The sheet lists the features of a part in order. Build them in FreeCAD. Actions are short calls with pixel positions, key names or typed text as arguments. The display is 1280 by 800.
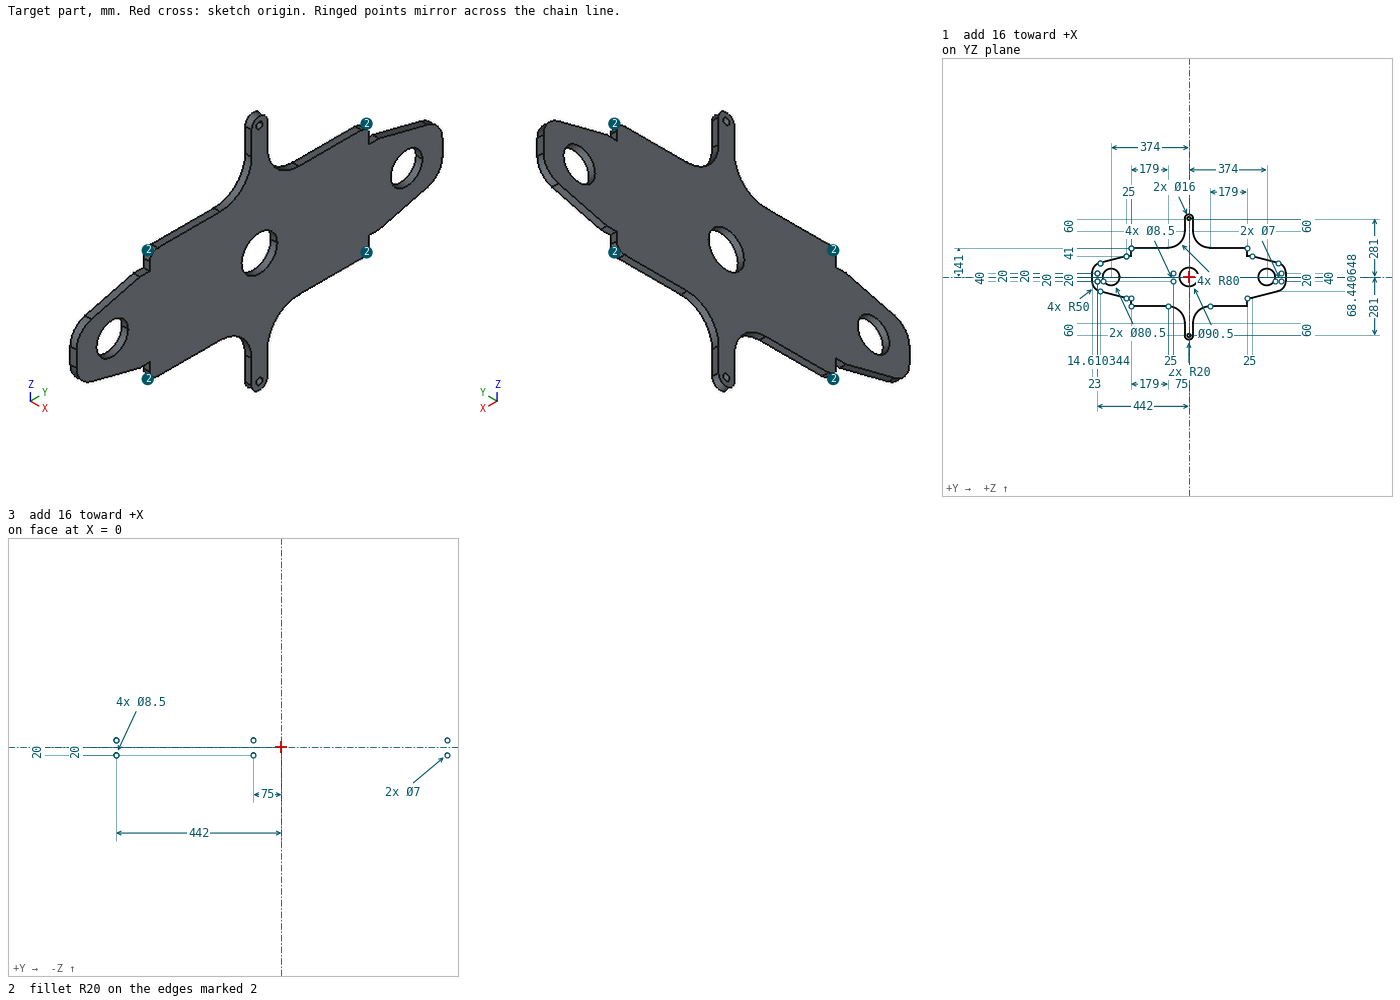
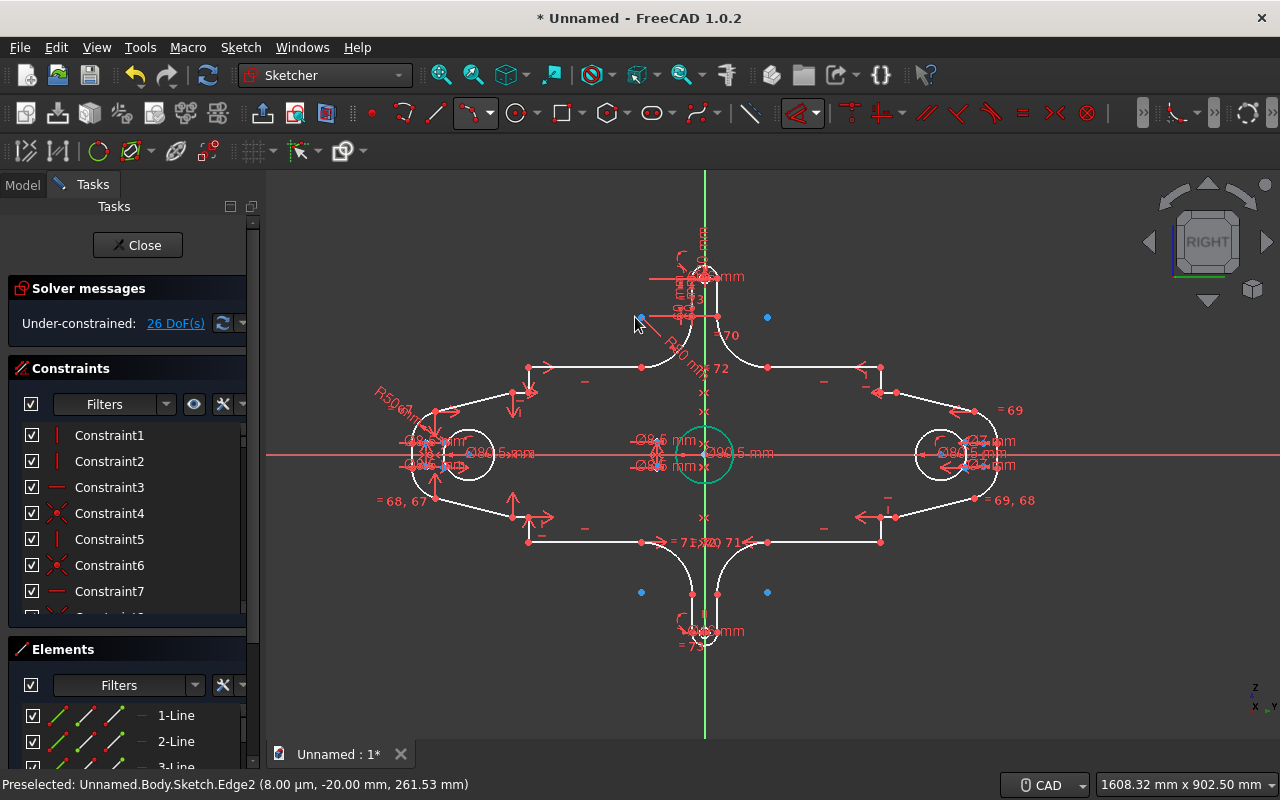
scroll(529, 375, up, 4)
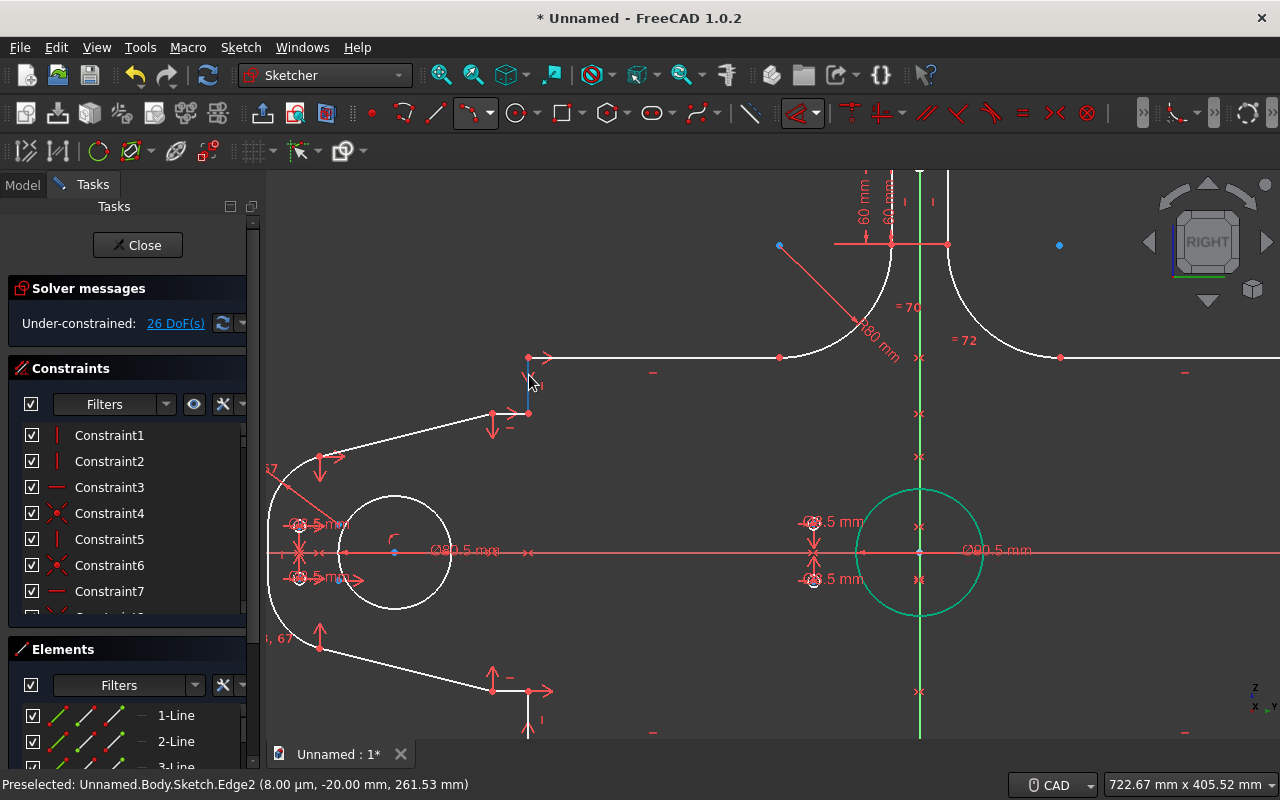
click(528, 375)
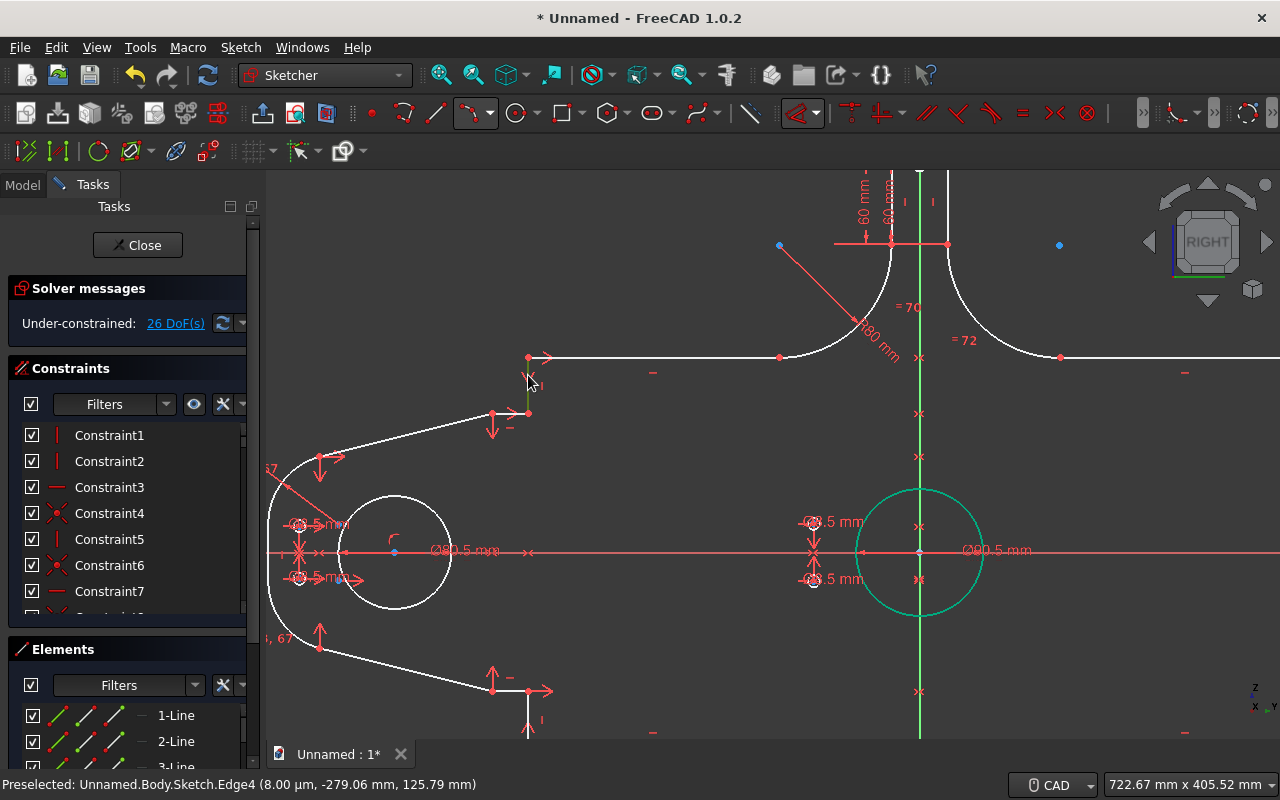
key(i)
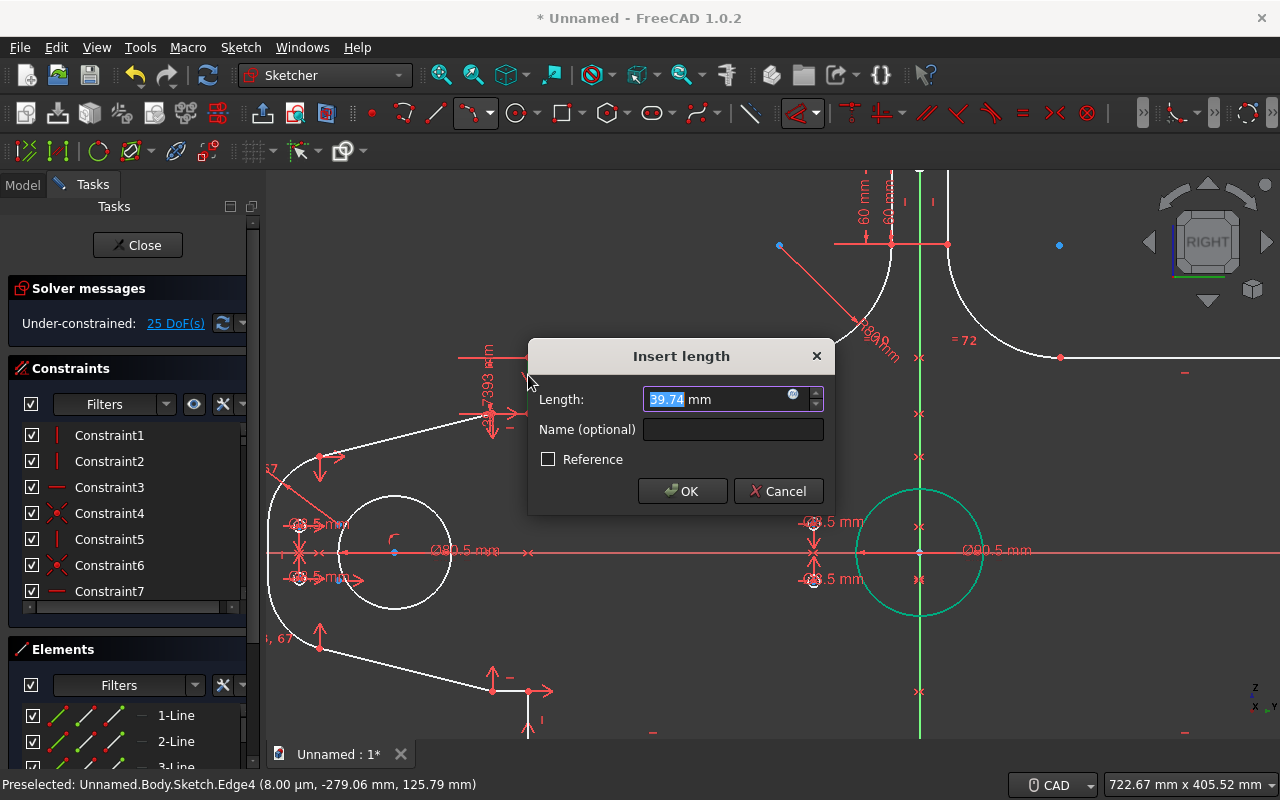
text(41)
key(Return)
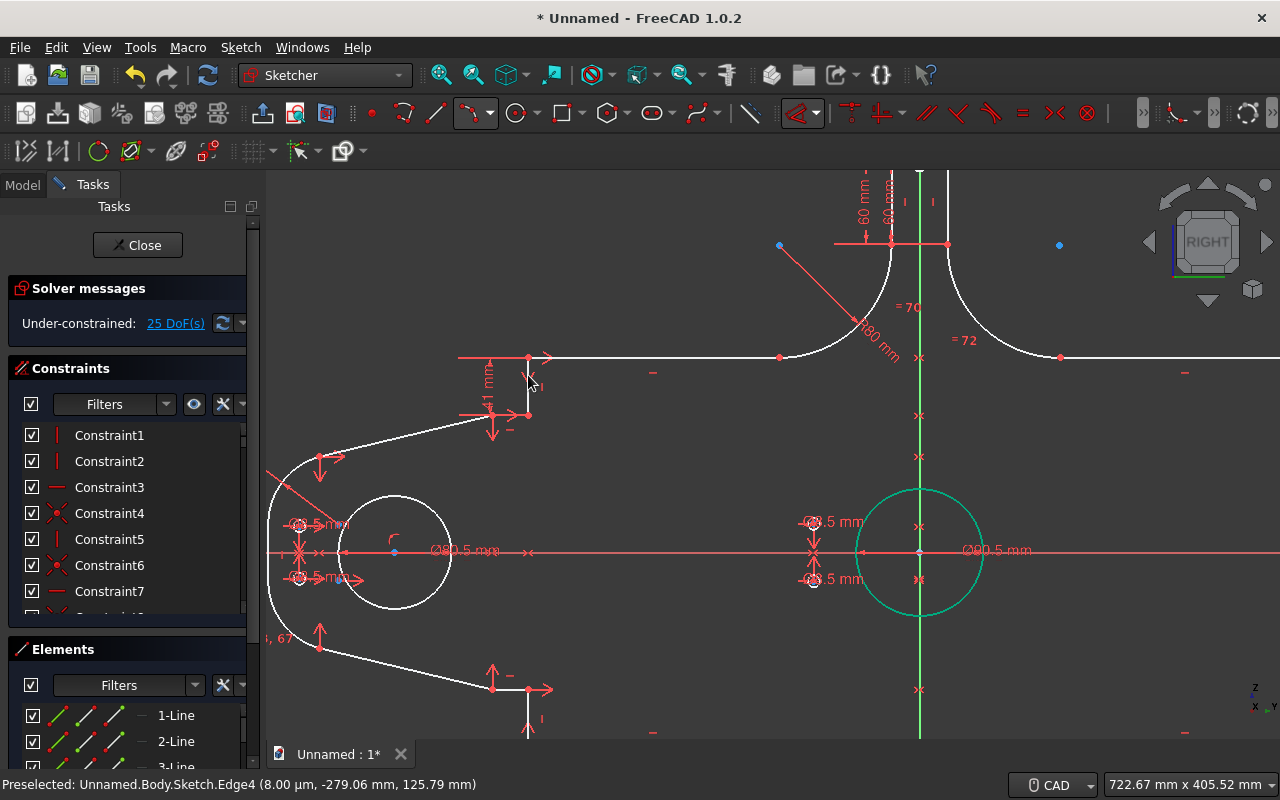
scroll(517, 415, up, 2)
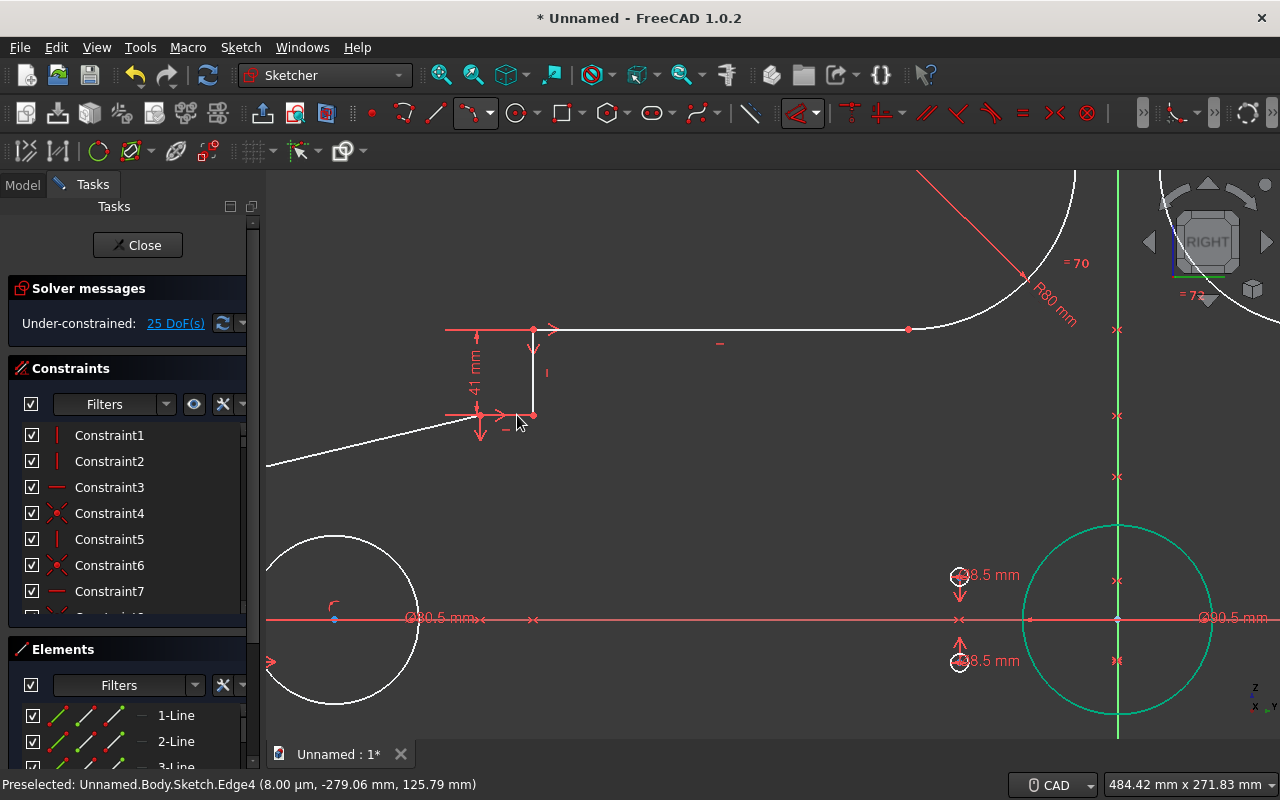
click(518, 415)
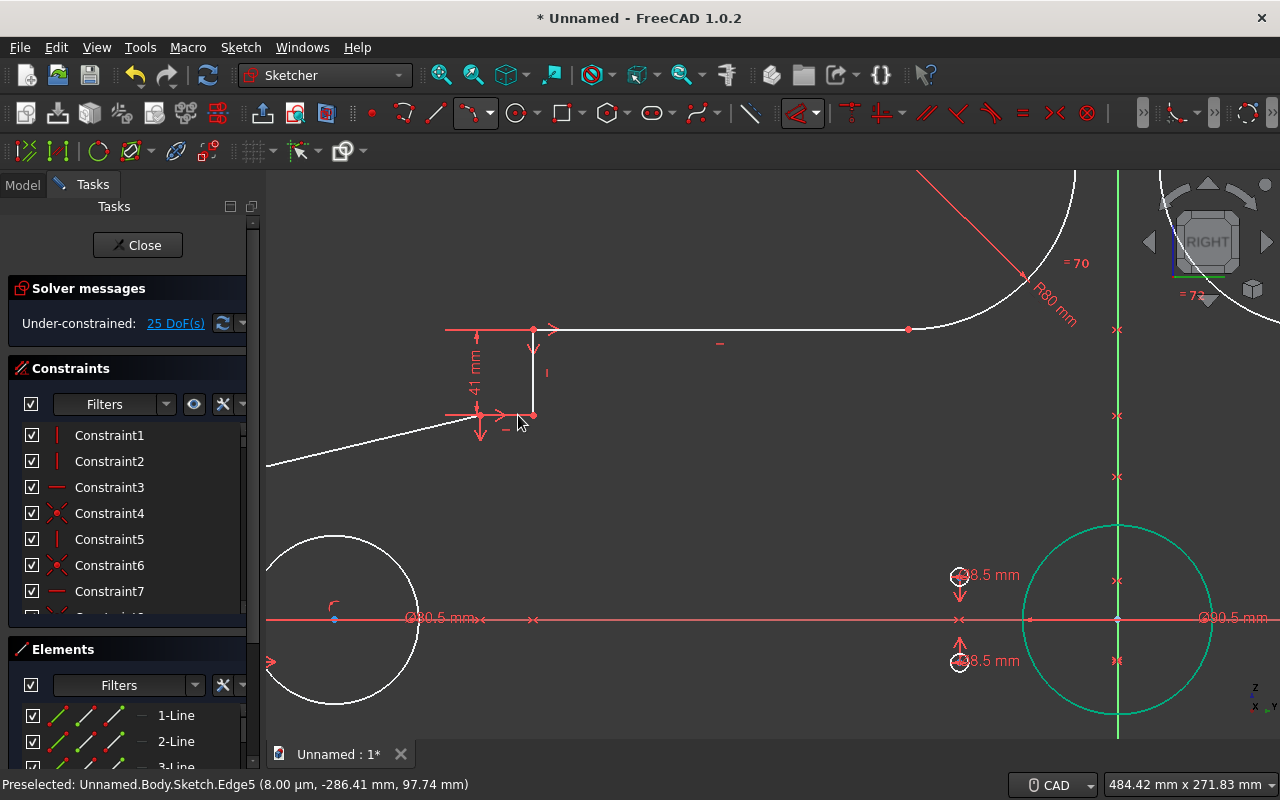
key(l)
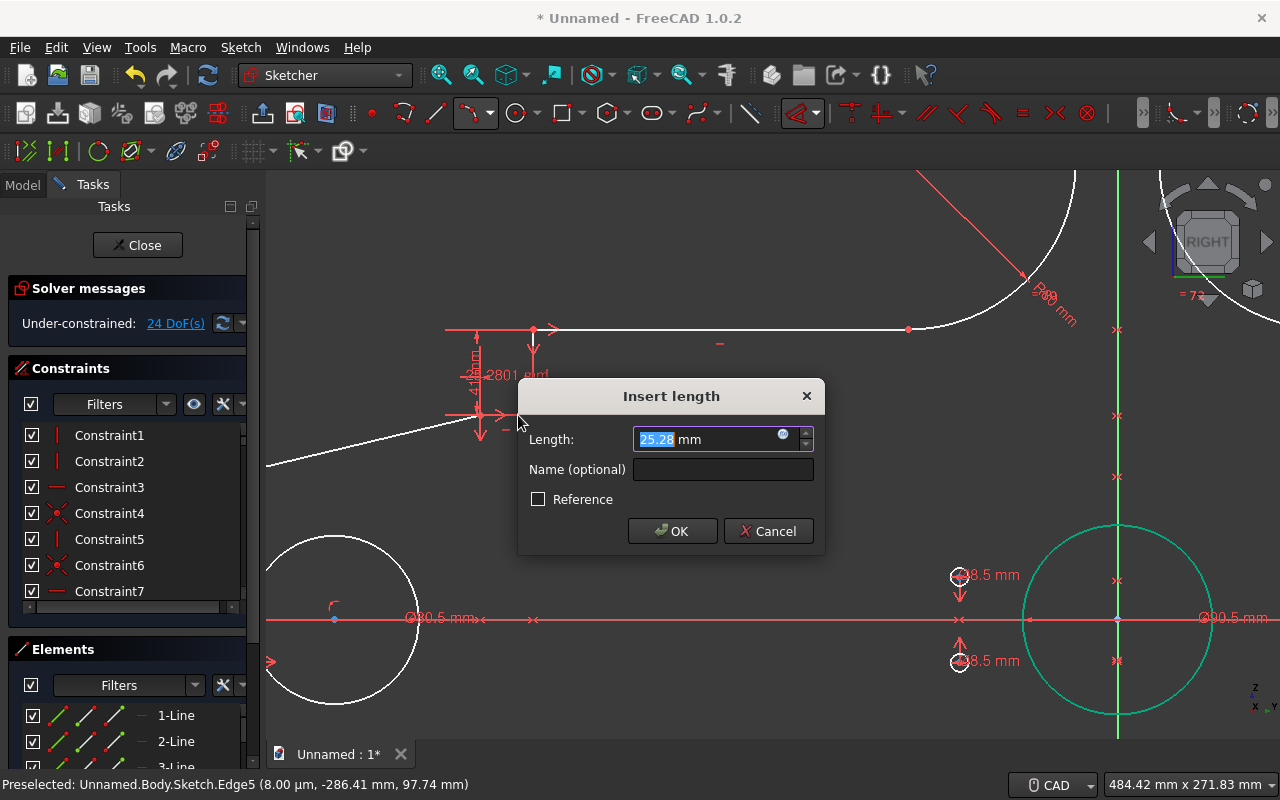
text(25)
key(Return)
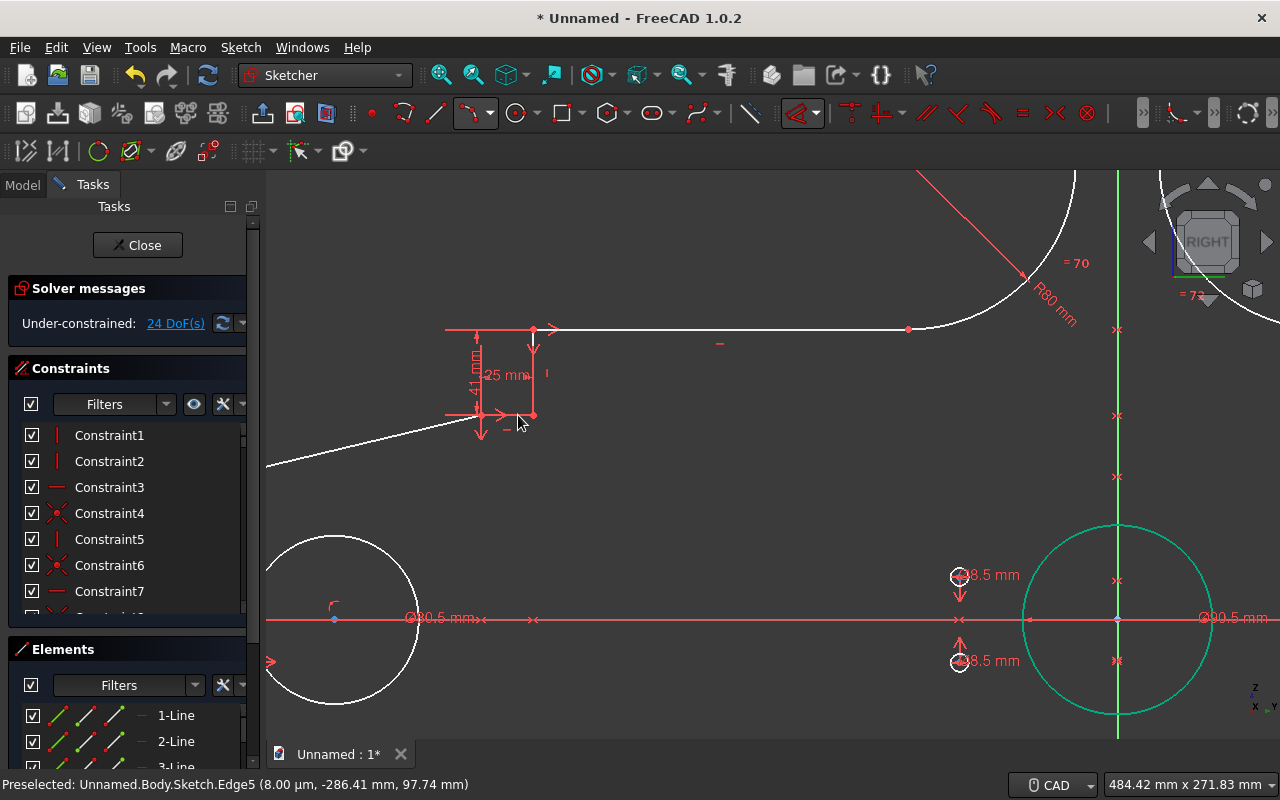
scroll(526, 383, down, 6)